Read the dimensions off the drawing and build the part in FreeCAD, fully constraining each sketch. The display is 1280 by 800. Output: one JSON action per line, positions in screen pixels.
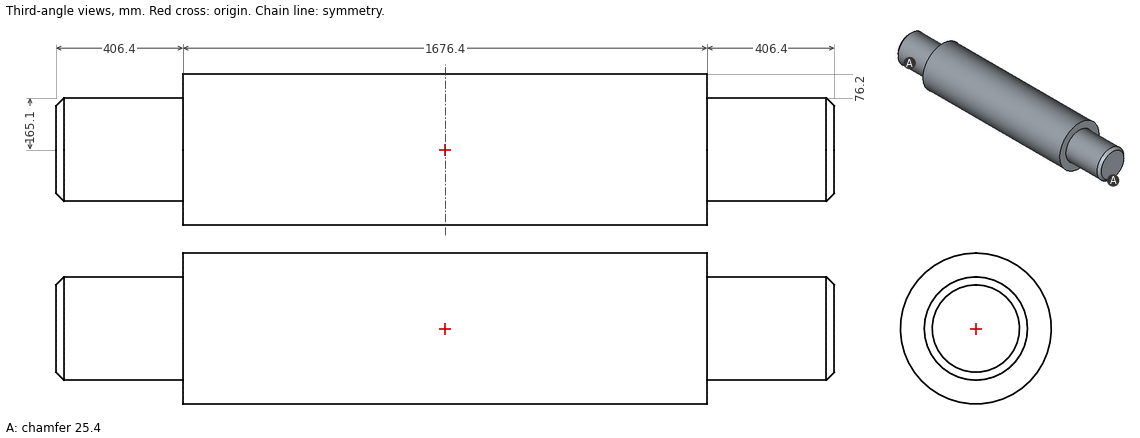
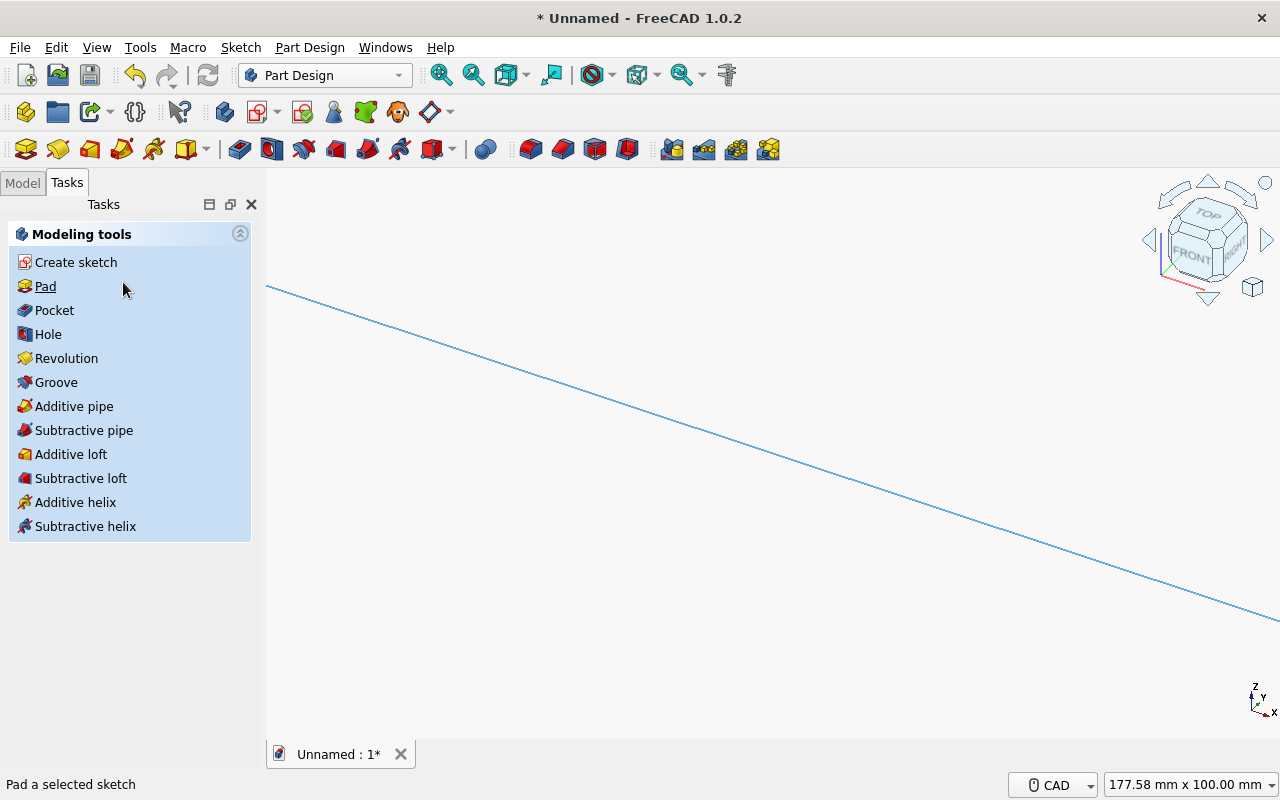
{"action": "left_click", "coordinate": [58, 150]}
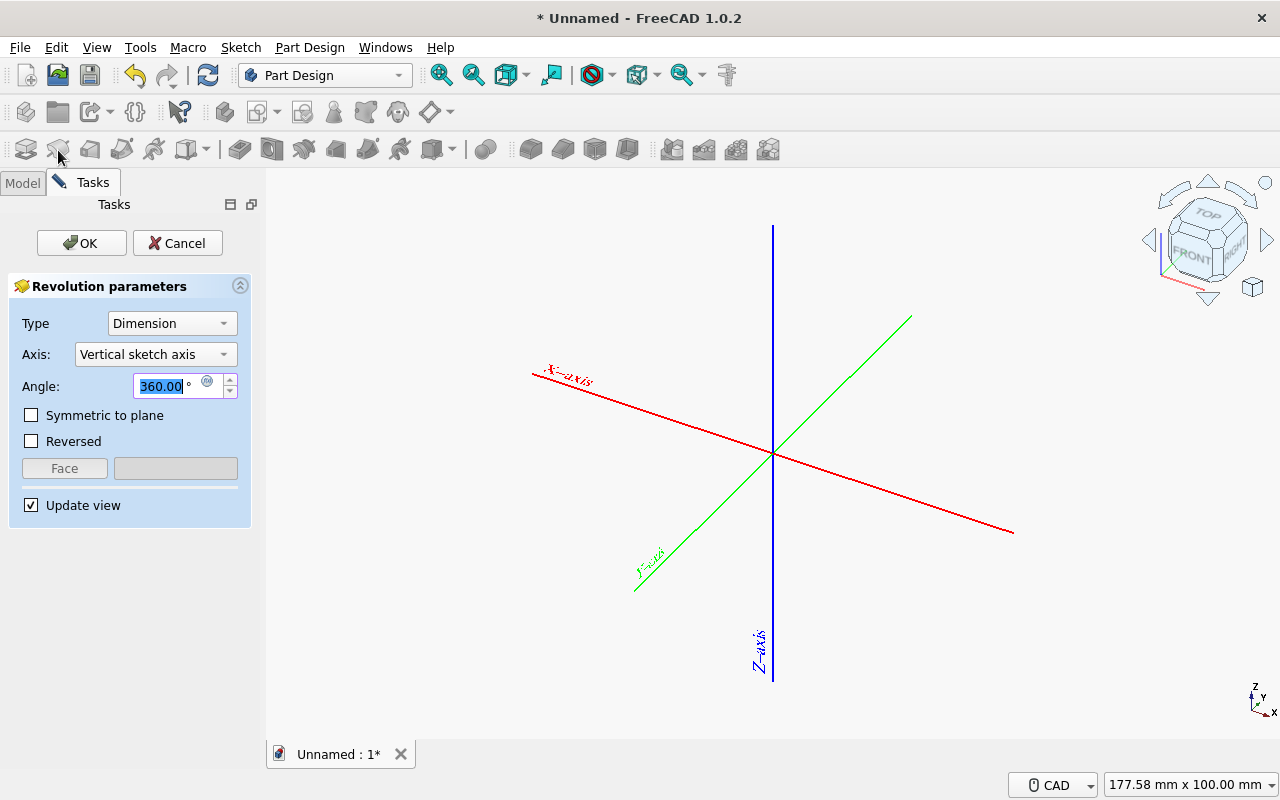
{"action": "left_click", "coordinate": [156, 354]}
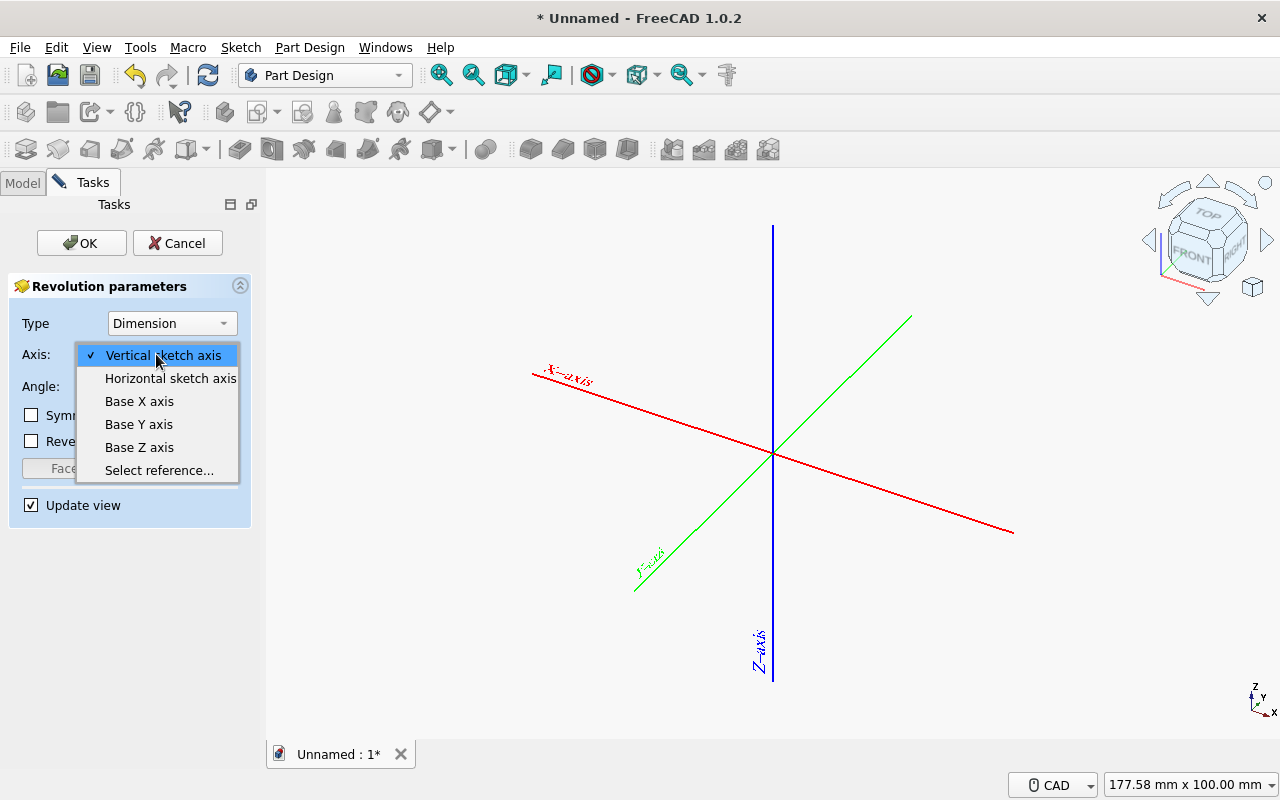
{"action": "left_click", "coordinate": [156, 378]}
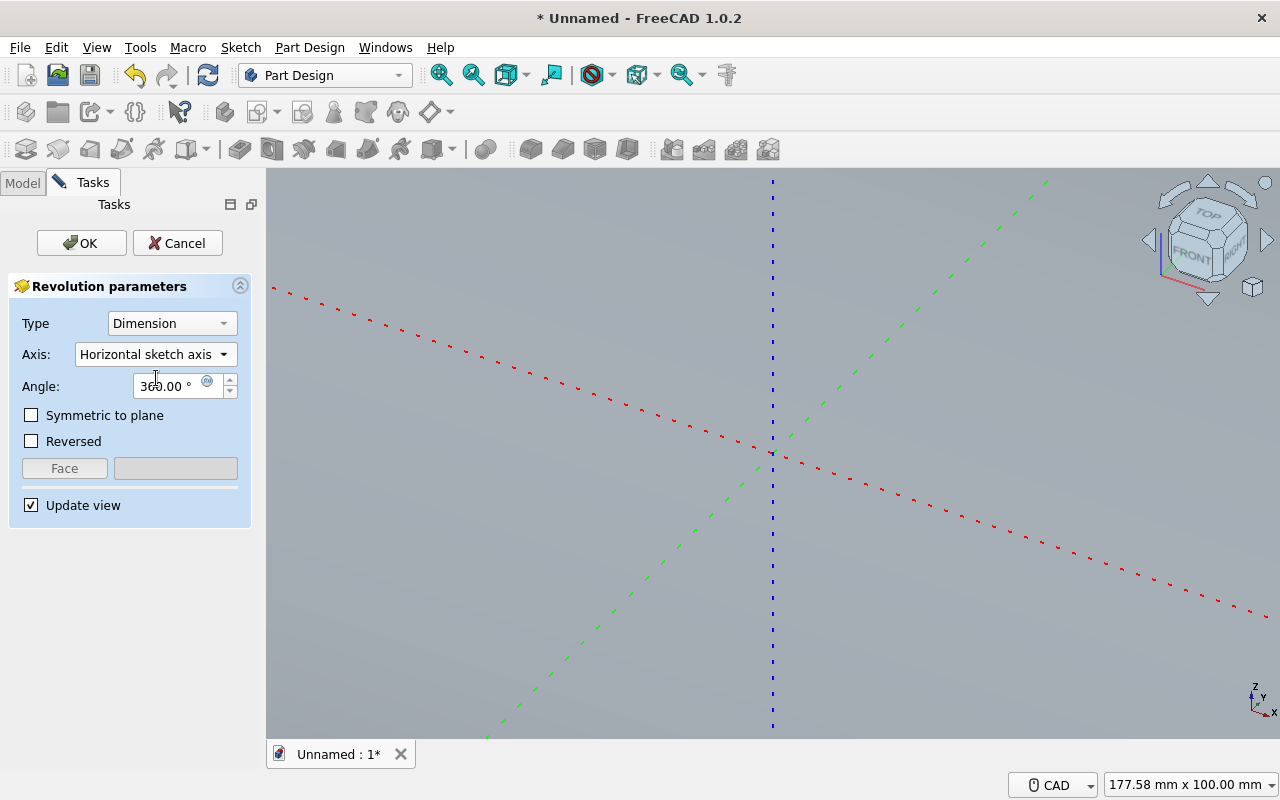
{"action": "left_click", "coordinate": [82, 243]}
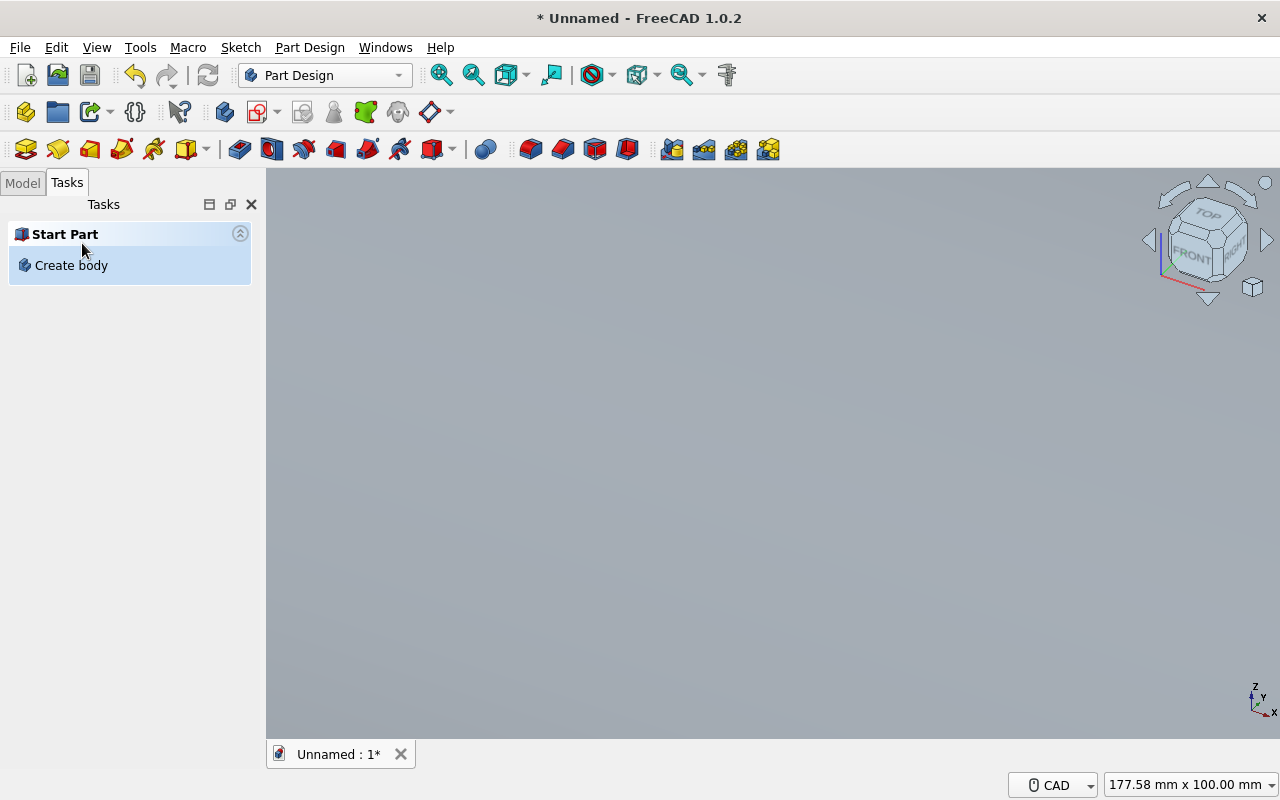
{"action": "key", "text": "v f"}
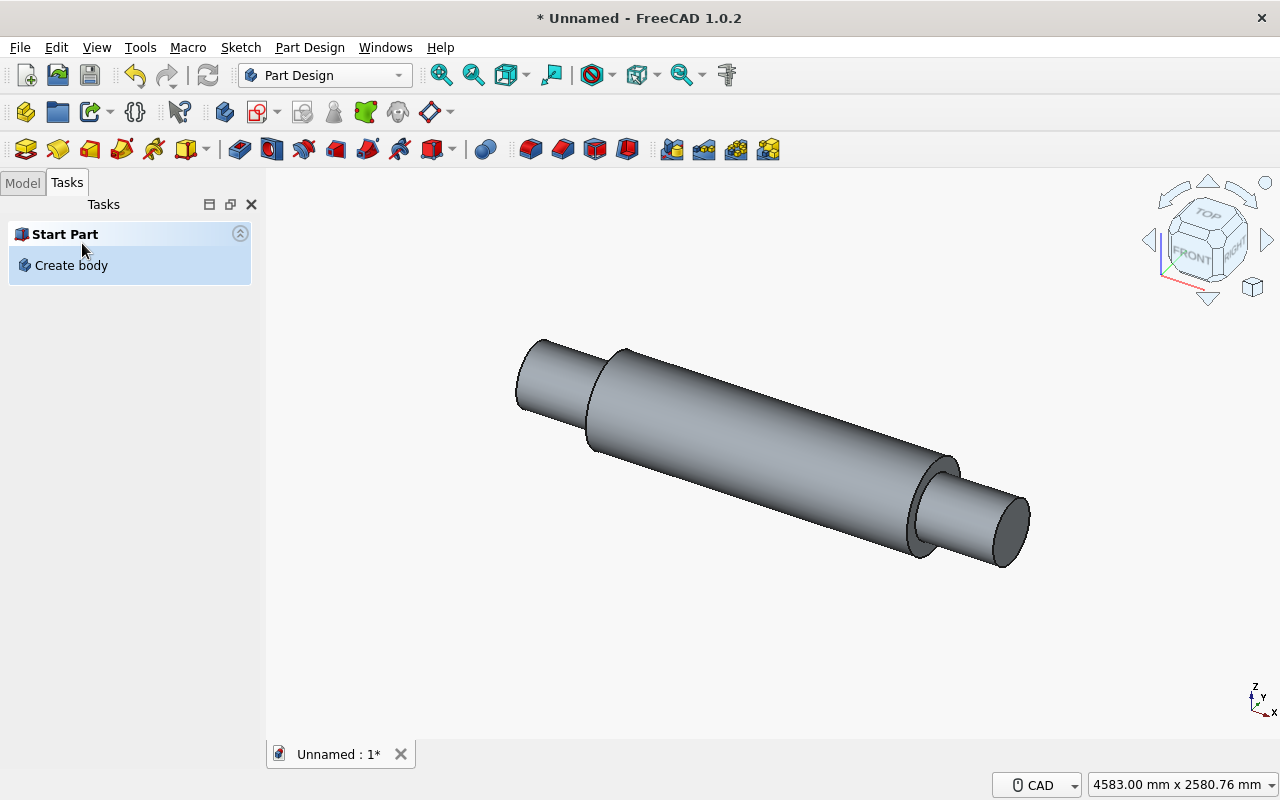
{"action": "left_click", "coordinate": [540, 340]}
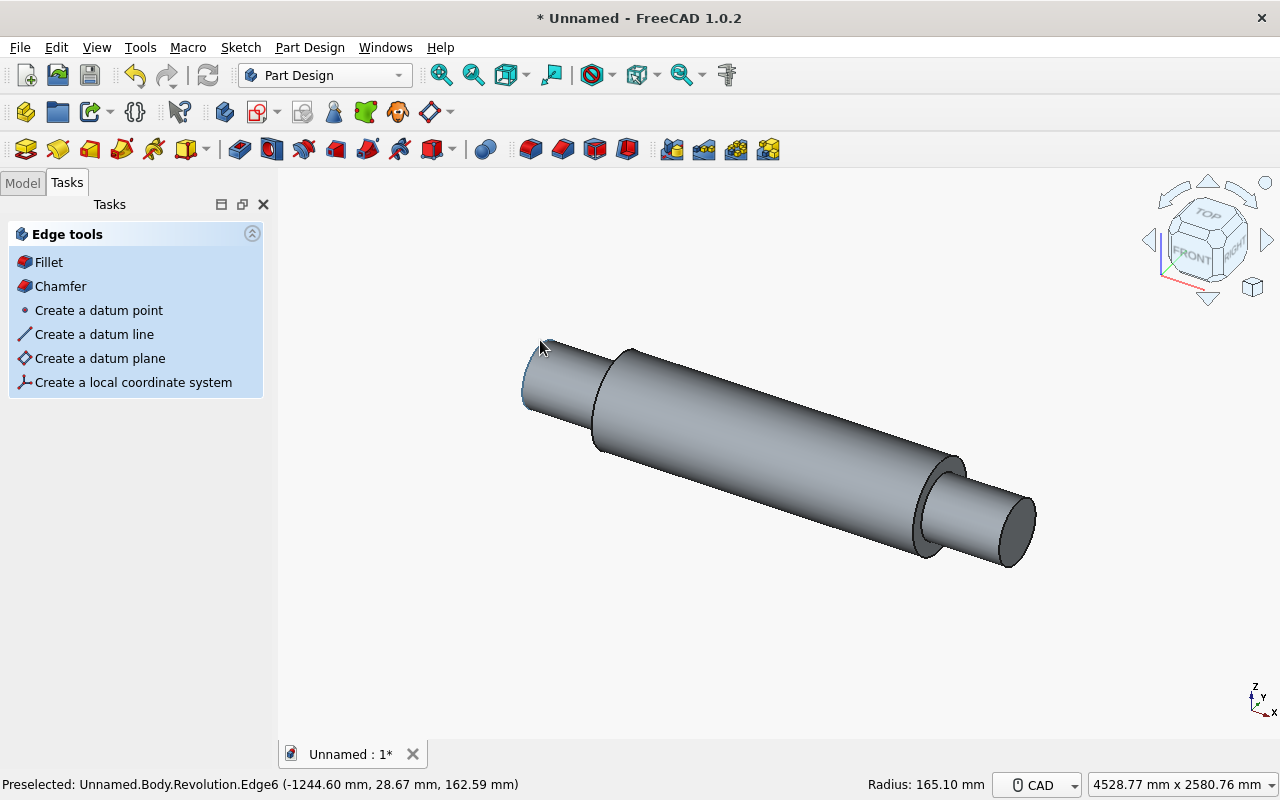
{"action": "left_click", "coordinate": [999, 550], "text": "ctrl"}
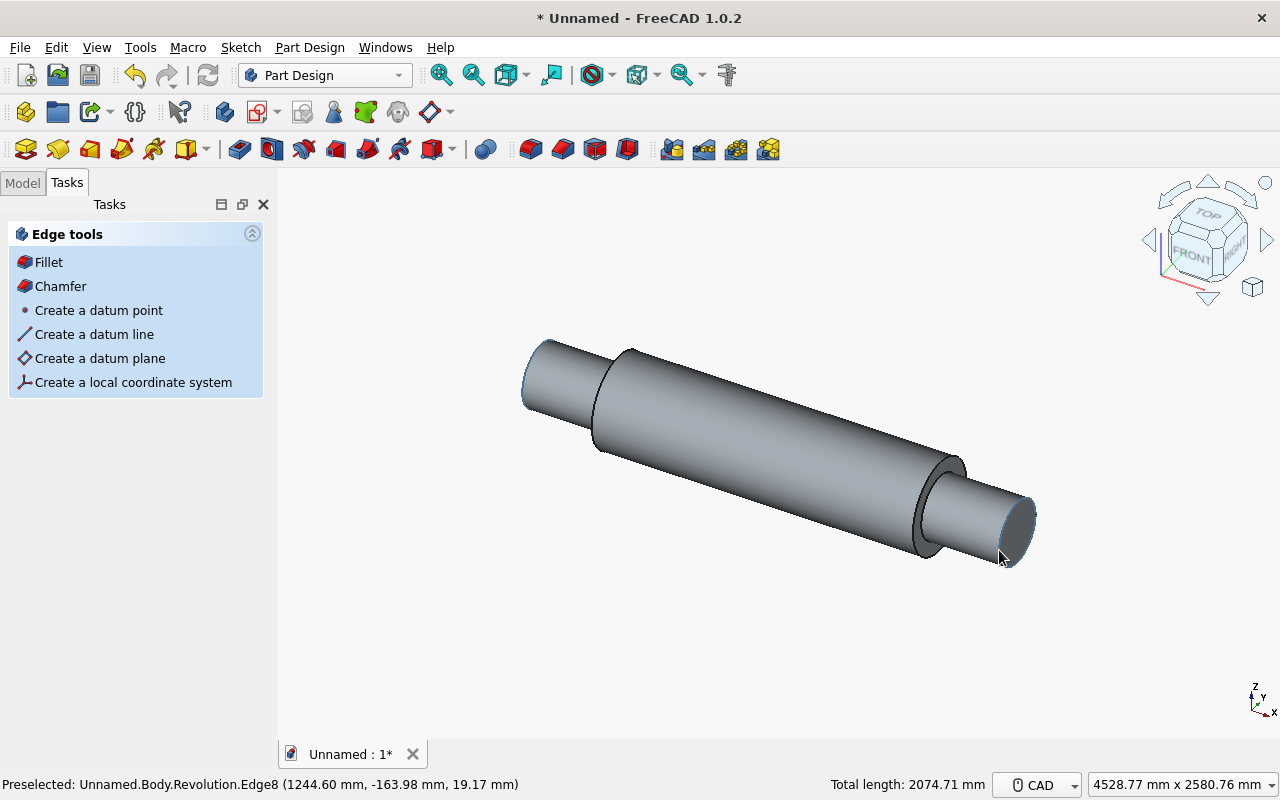
{"action": "left_click", "coordinate": [564, 150]}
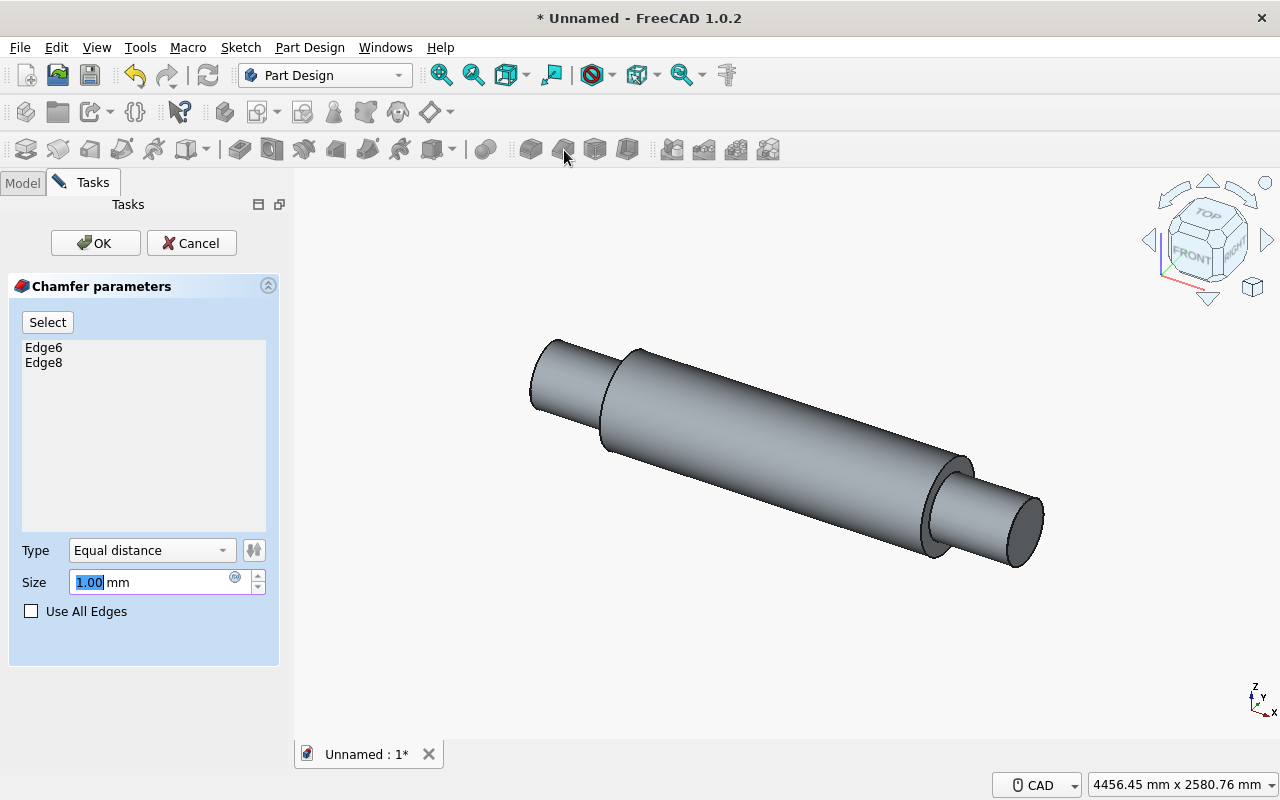
{"action": "type", "text": "25.4"}
{"action": "key", "text": "Tab"}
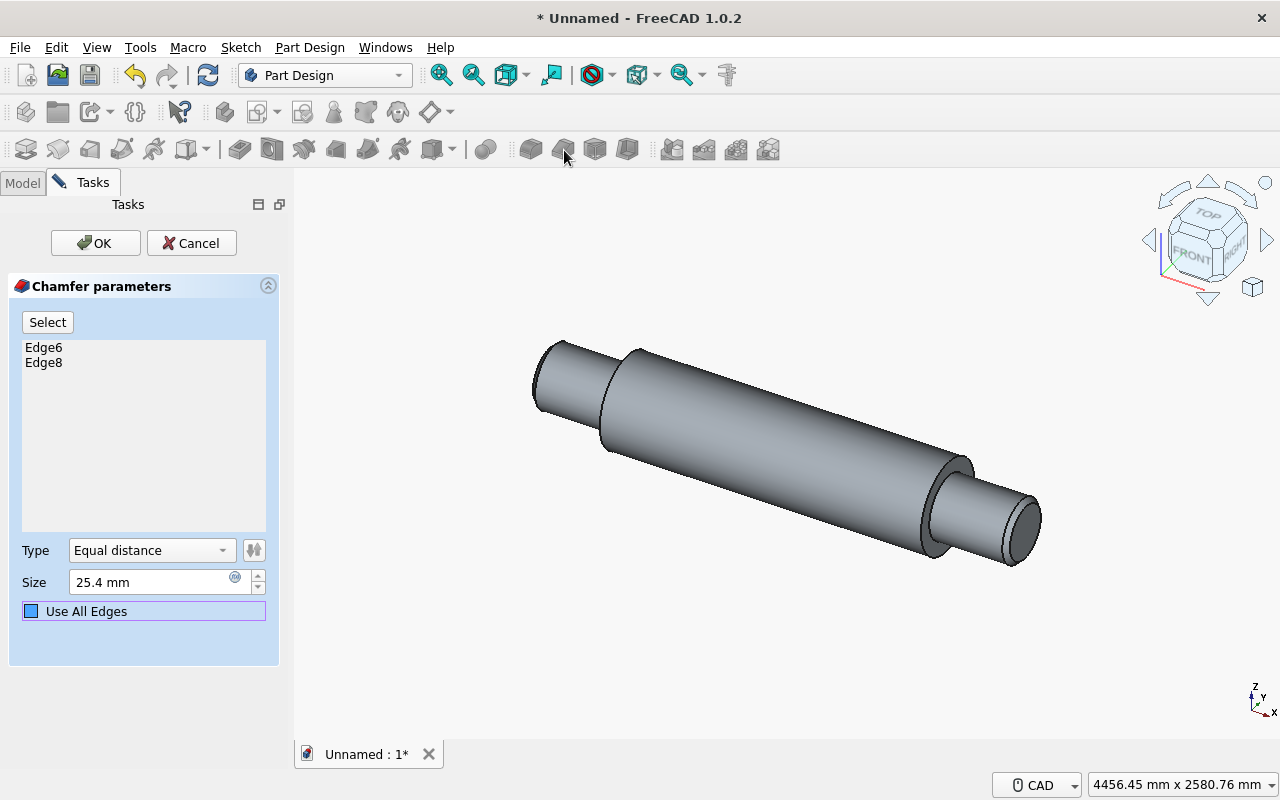
{"action": "left_click", "coordinate": [96, 243]}